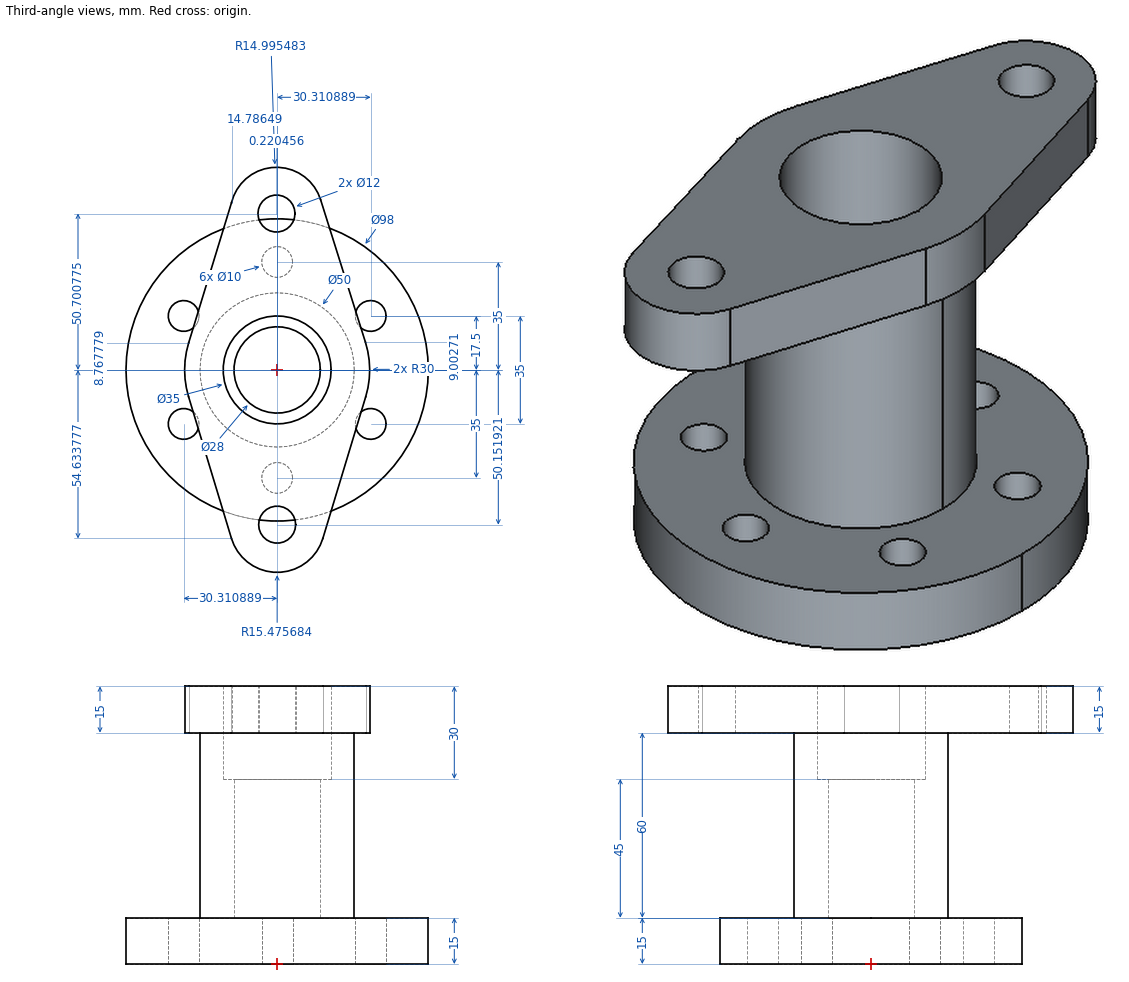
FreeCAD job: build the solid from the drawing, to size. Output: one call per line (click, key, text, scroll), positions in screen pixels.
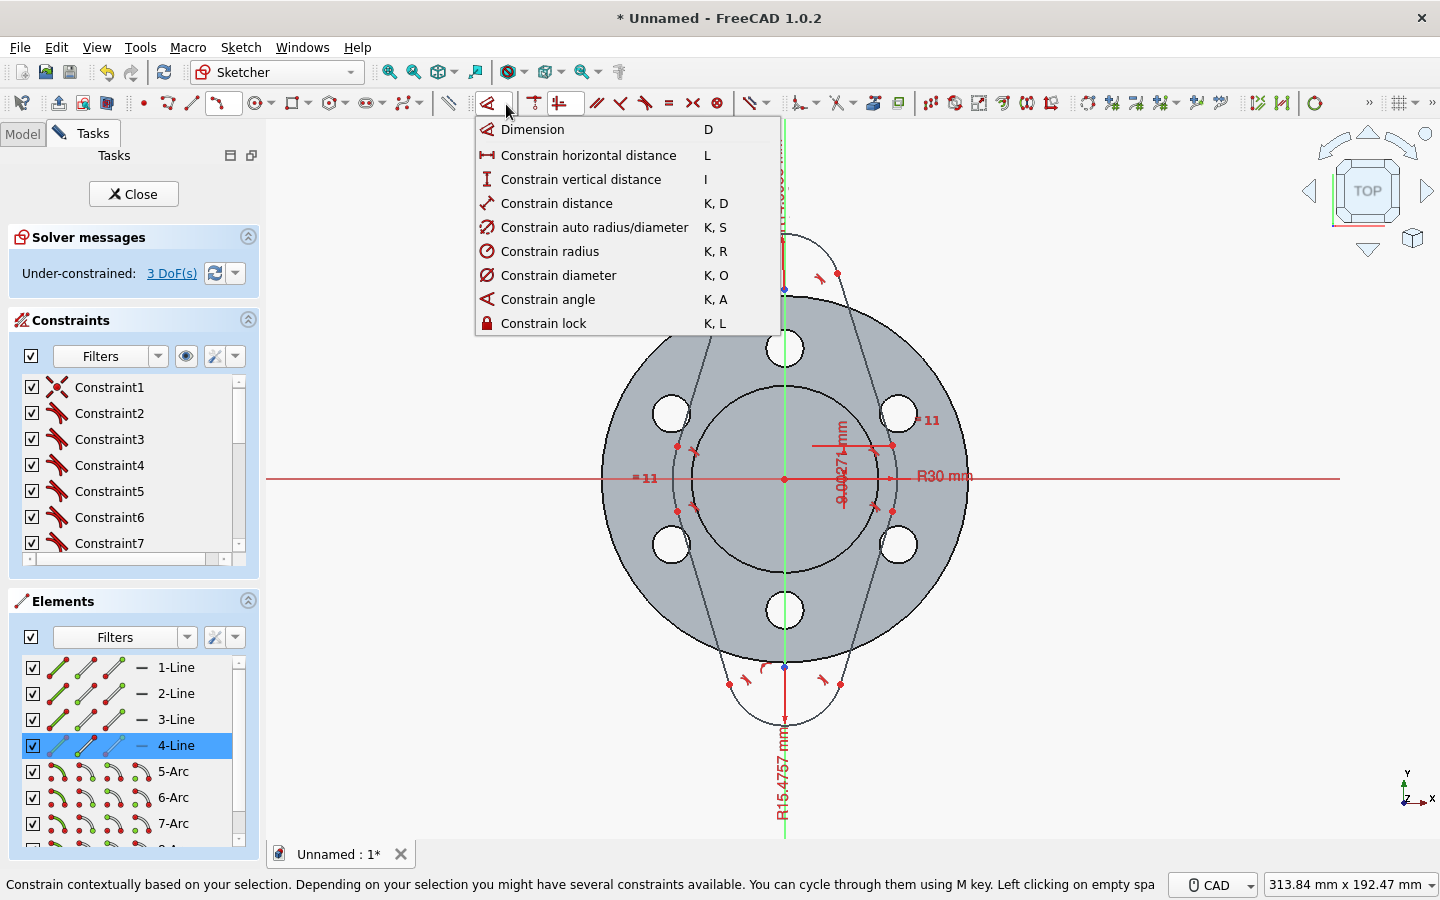
click(628, 155)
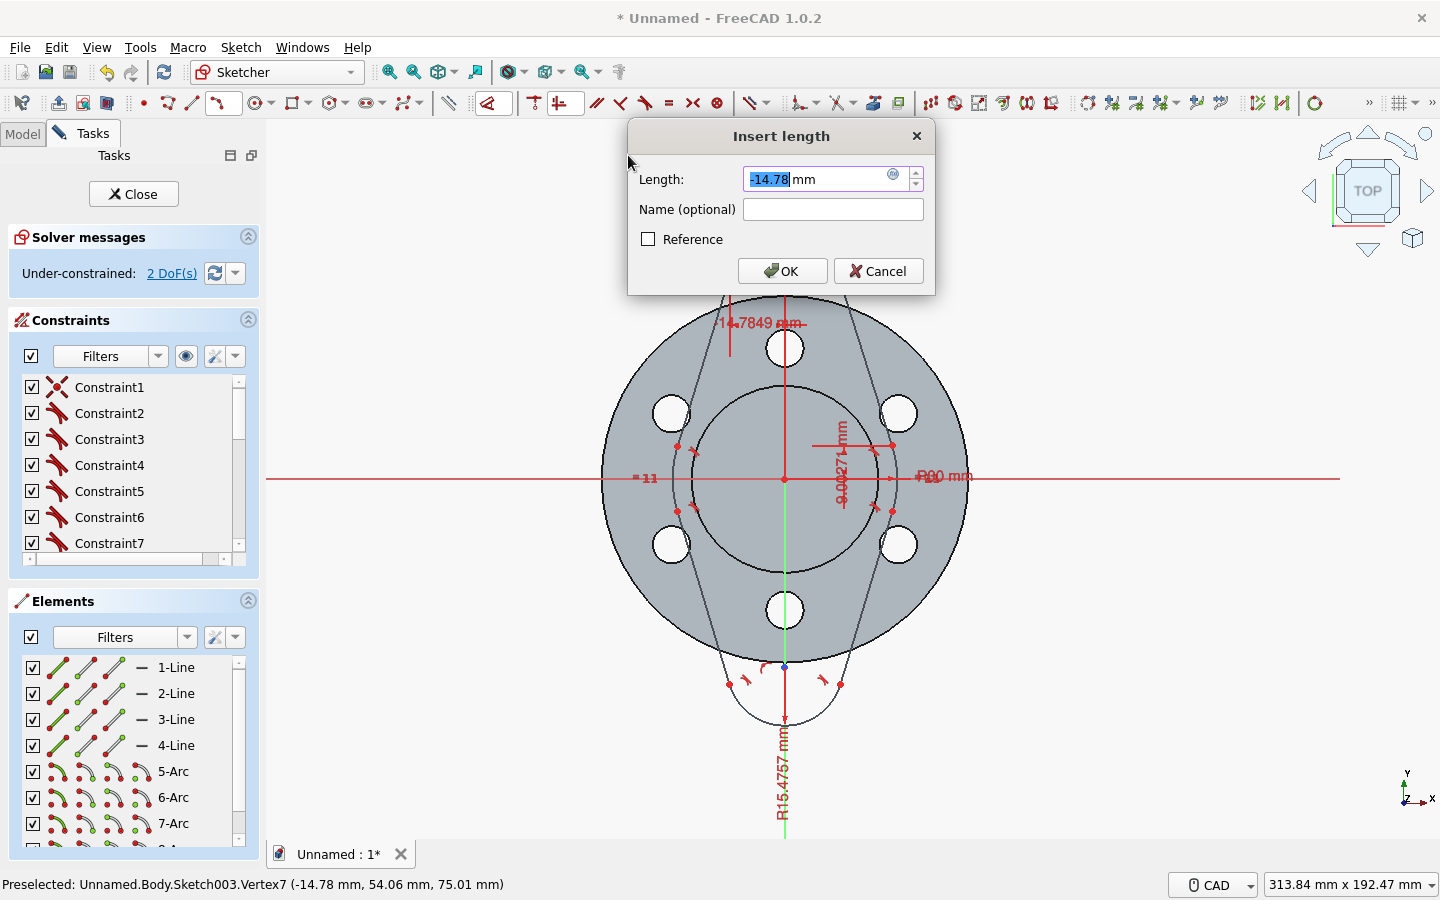
text(-14.78649)
key(Return)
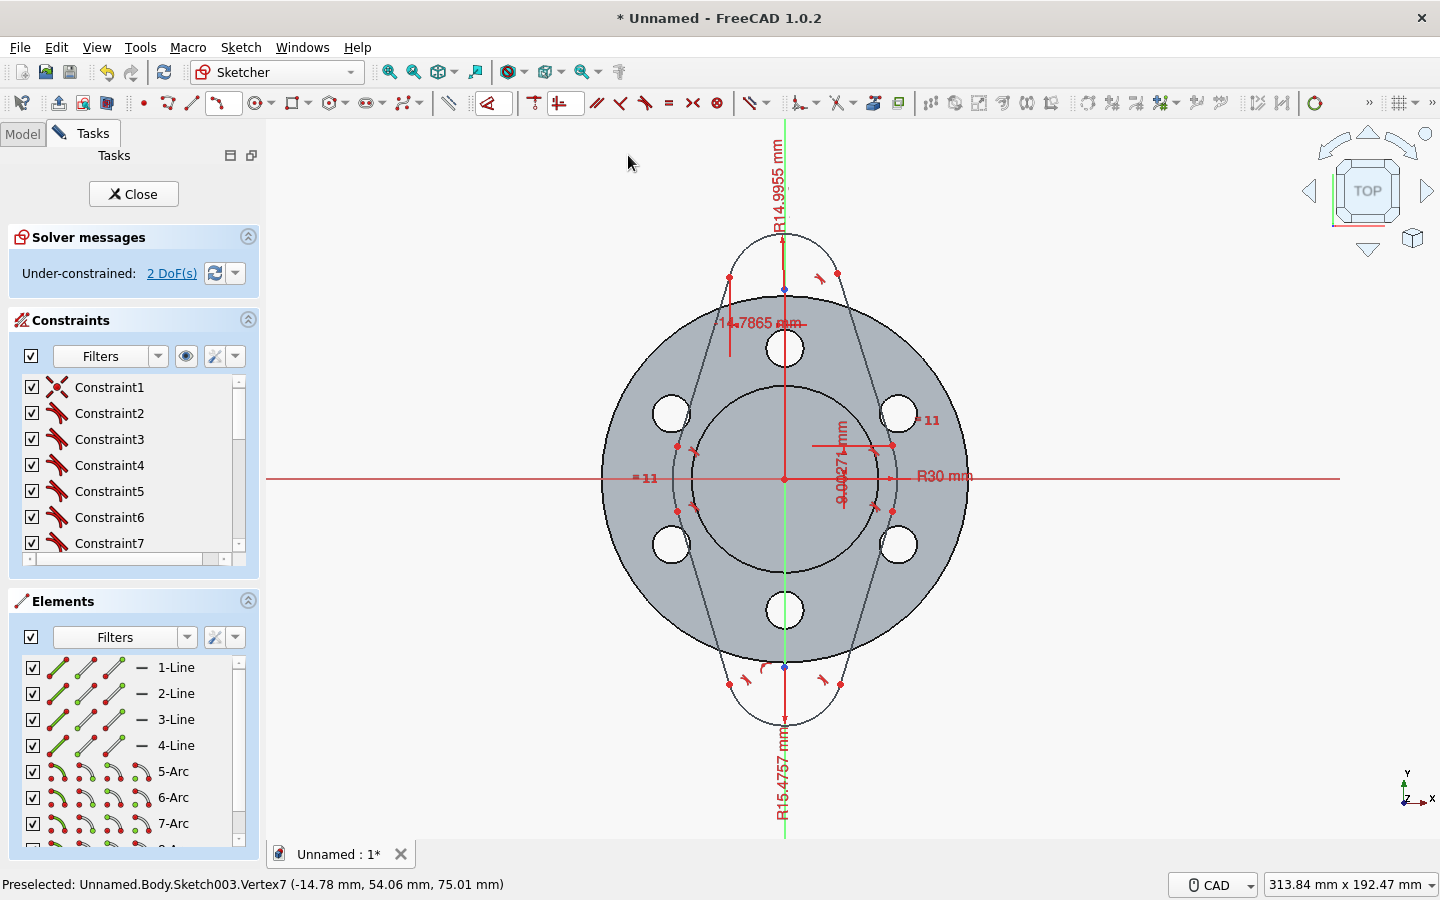
click(678, 446)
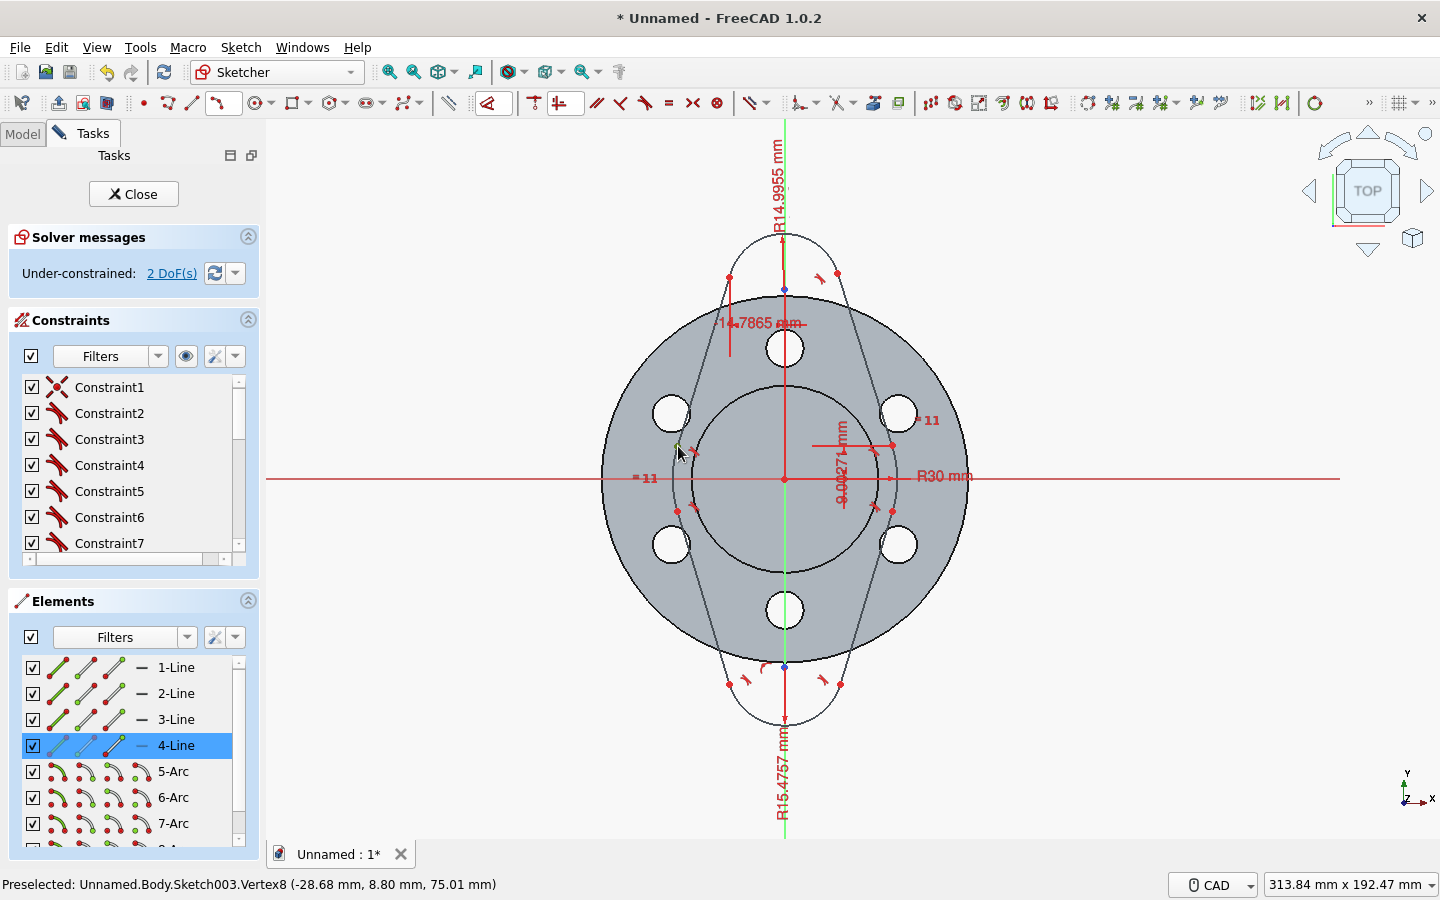
key(i)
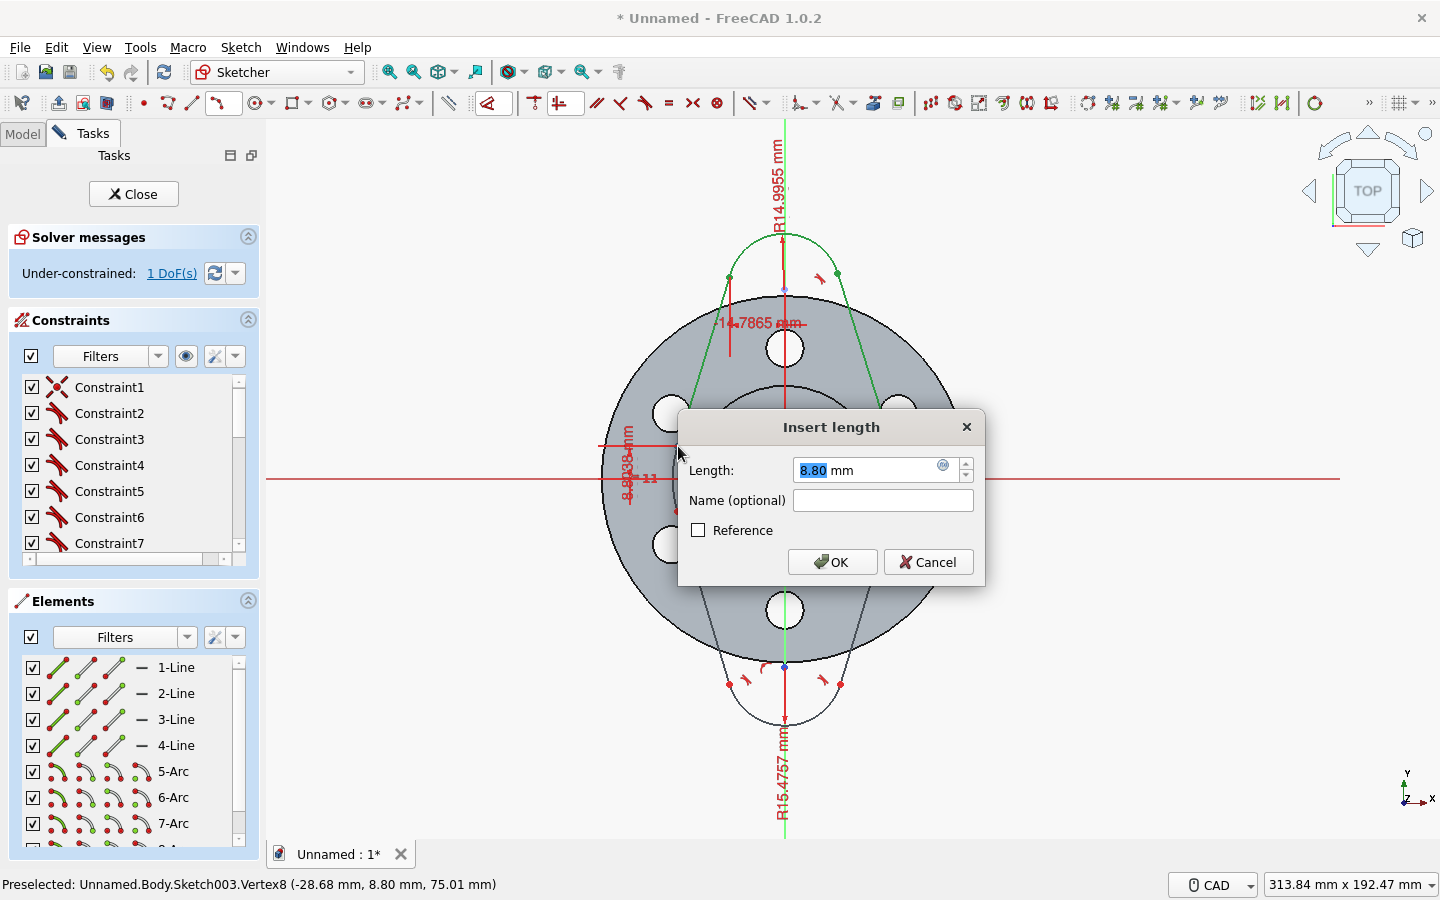
text(8.767779)
key(Return)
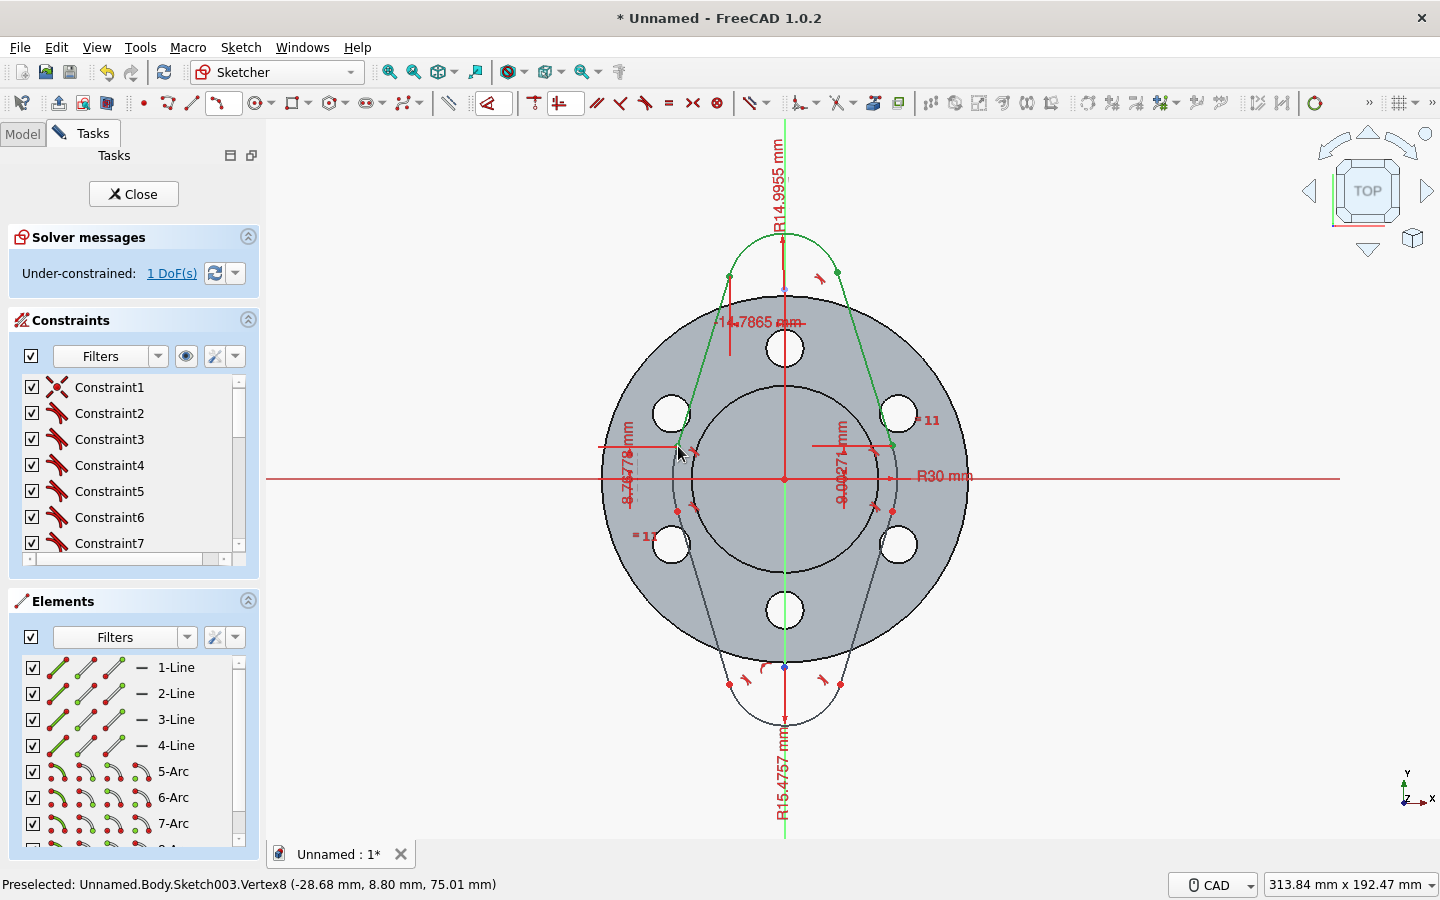
click(730, 684)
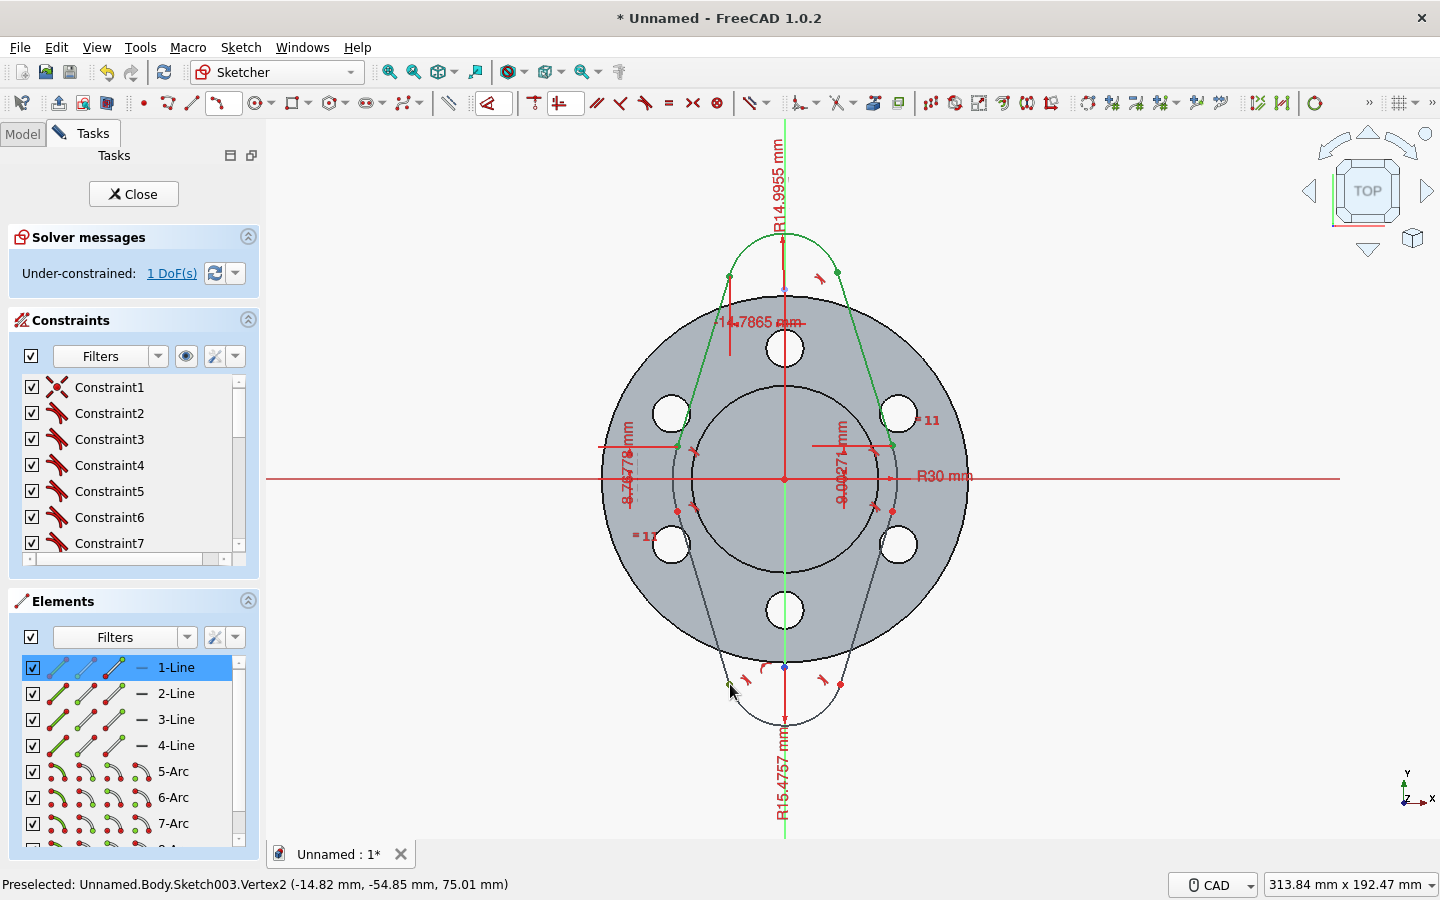
key(i)